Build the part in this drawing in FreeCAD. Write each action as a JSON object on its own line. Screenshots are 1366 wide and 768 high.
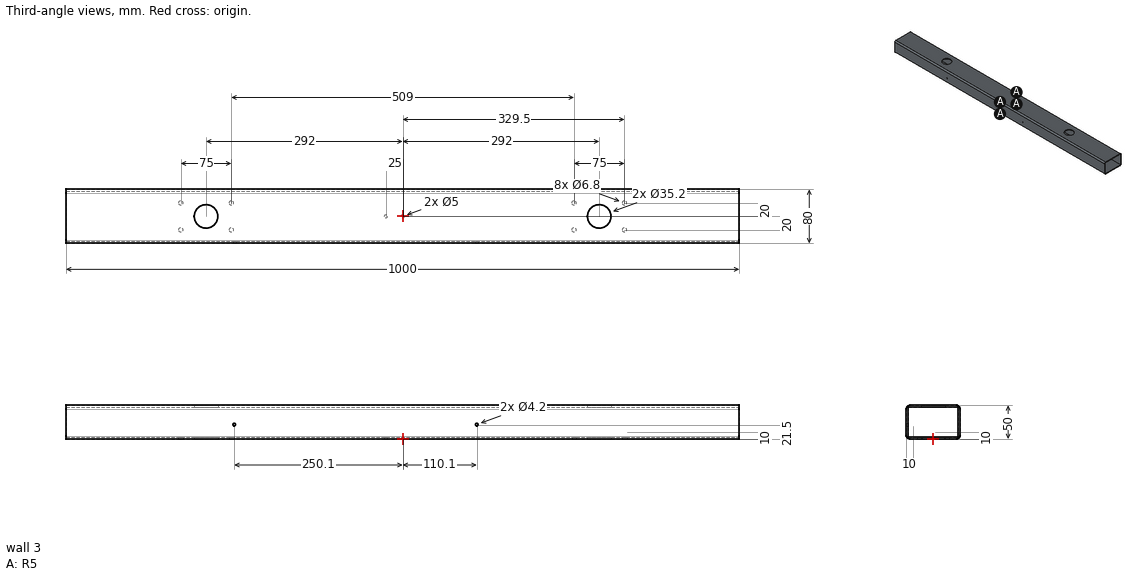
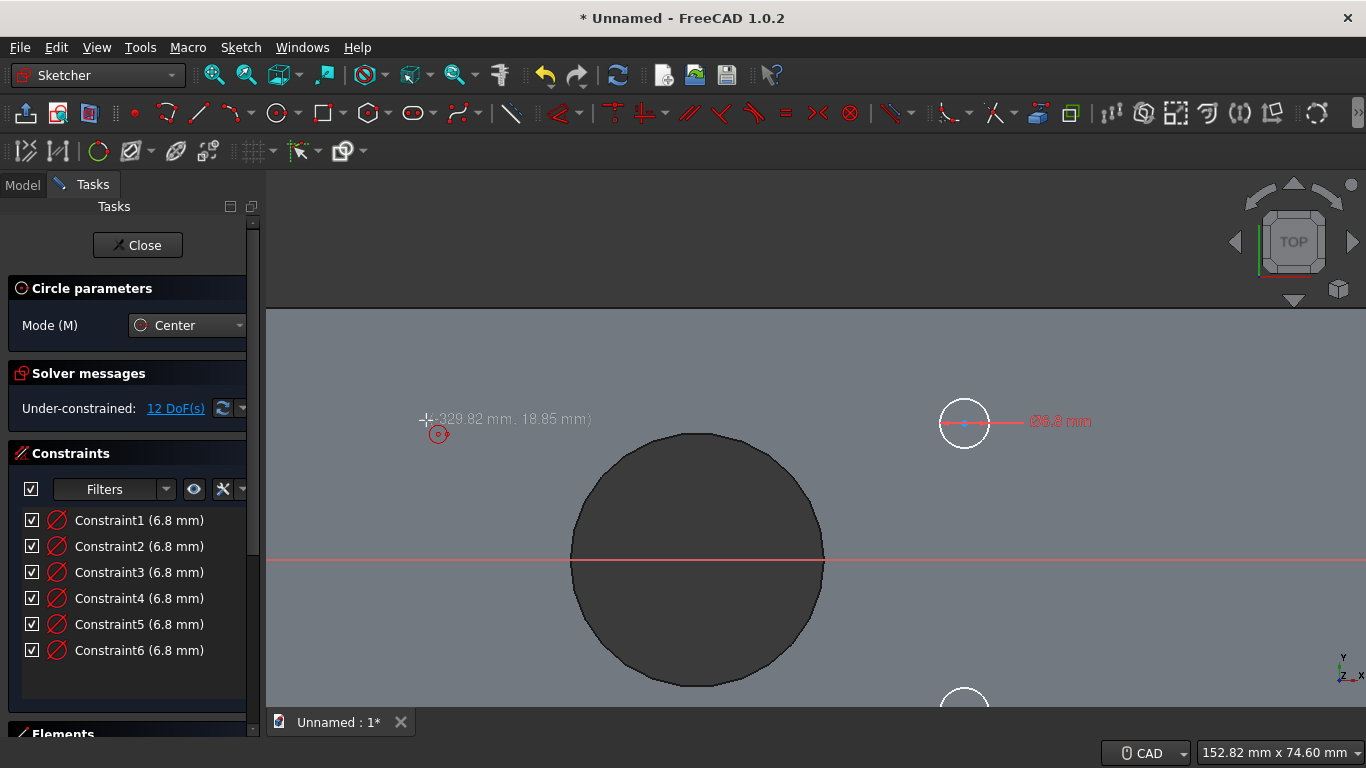
{"action": "scroll", "coordinate": [426, 419], "scroll_direction": "down", "scroll_amount": 10}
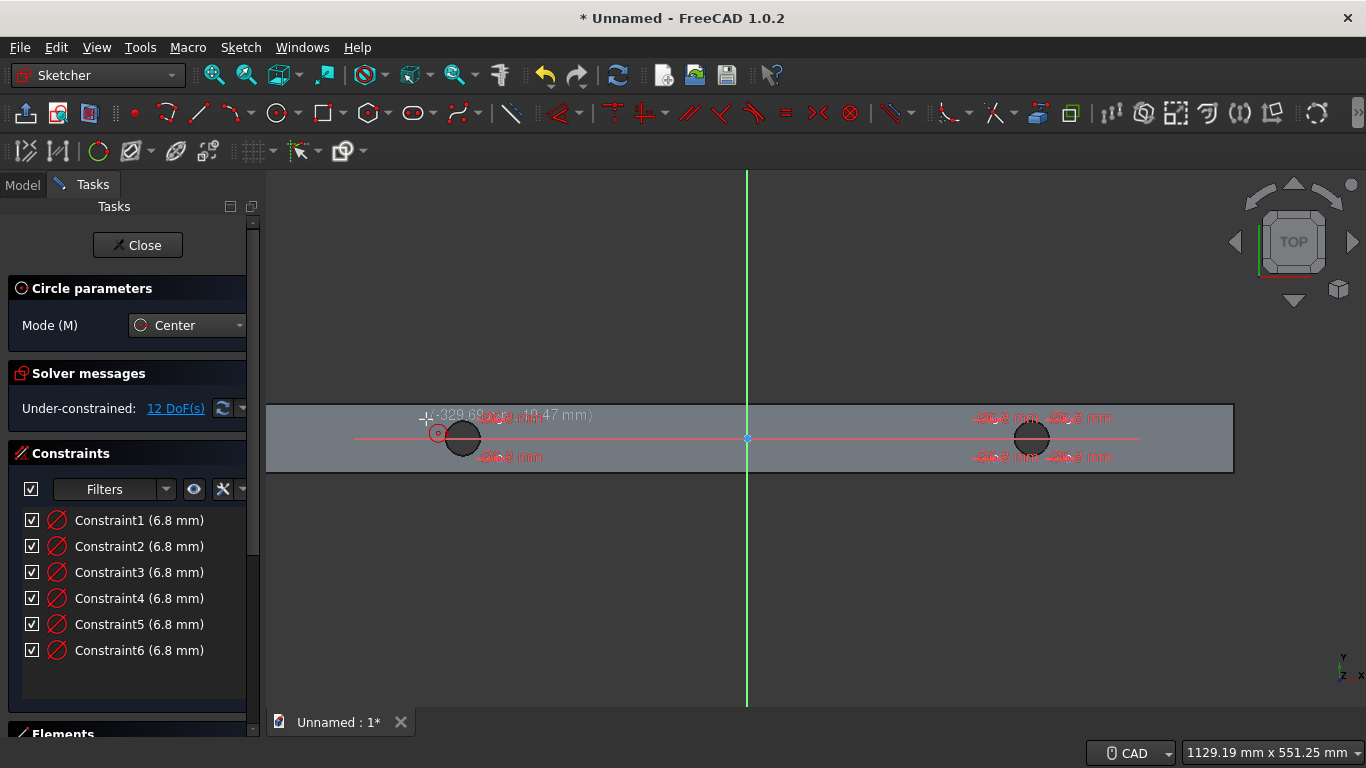
{"action": "left_click", "coordinate": [426, 419]}
{"action": "mouse_move", "coordinate": [429, 417]}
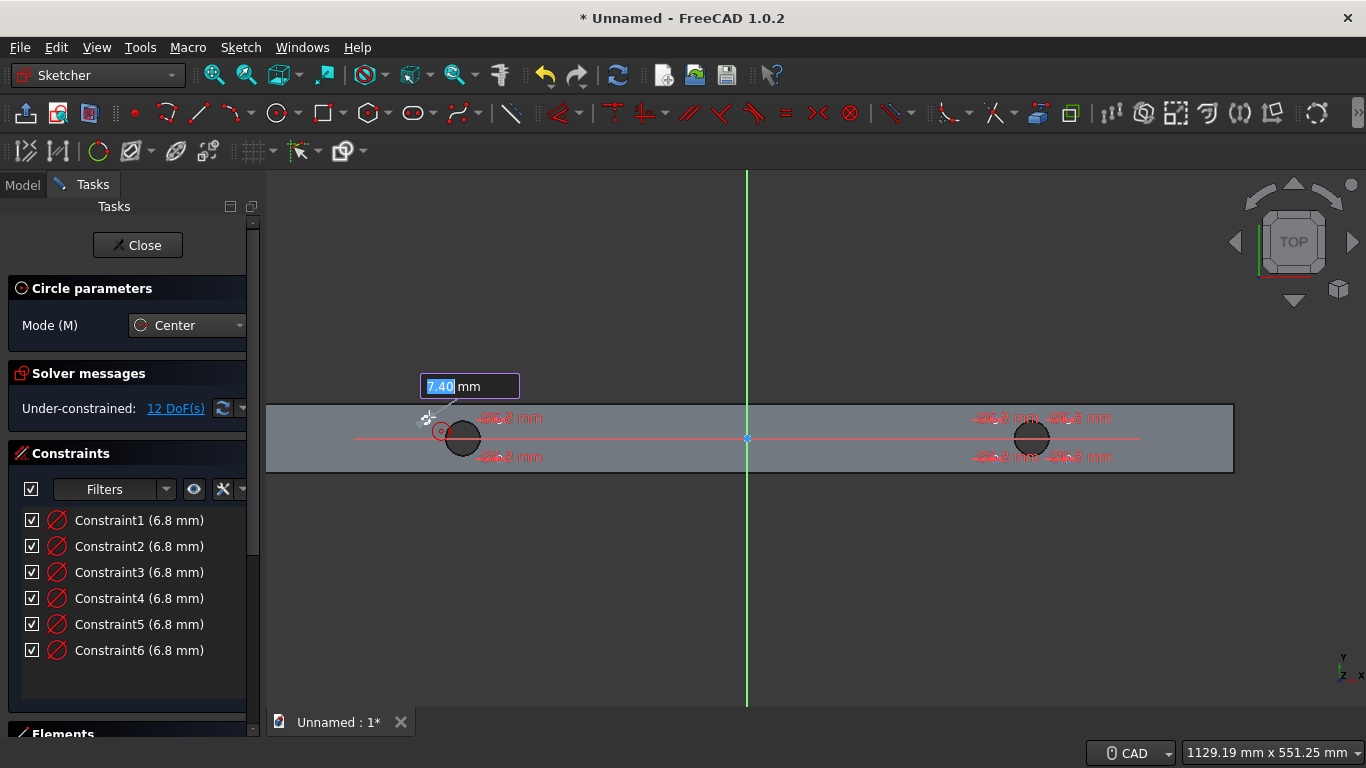
{"action": "type", "text": "6.8"}
{"action": "key", "text": "Return"}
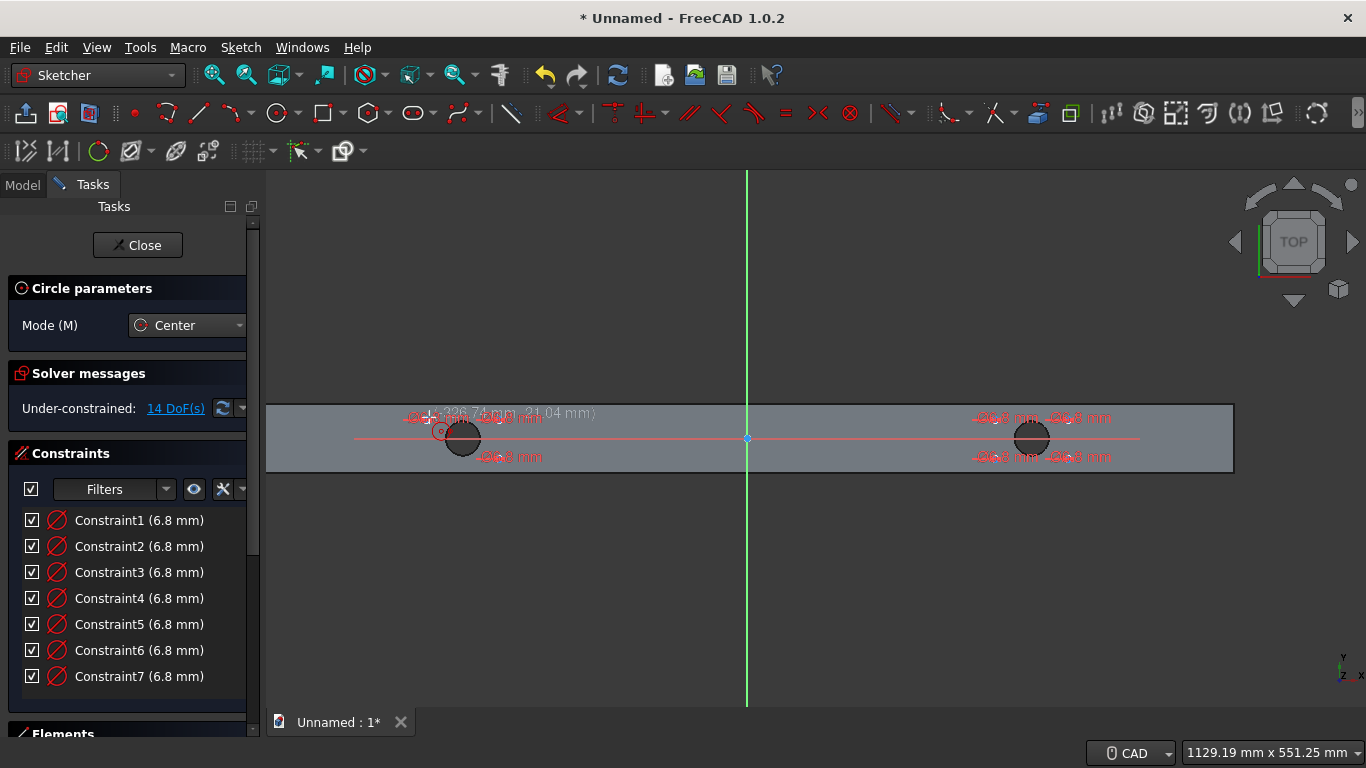
{"action": "scroll", "coordinate": [426, 458], "scroll_direction": "up", "scroll_amount": 10}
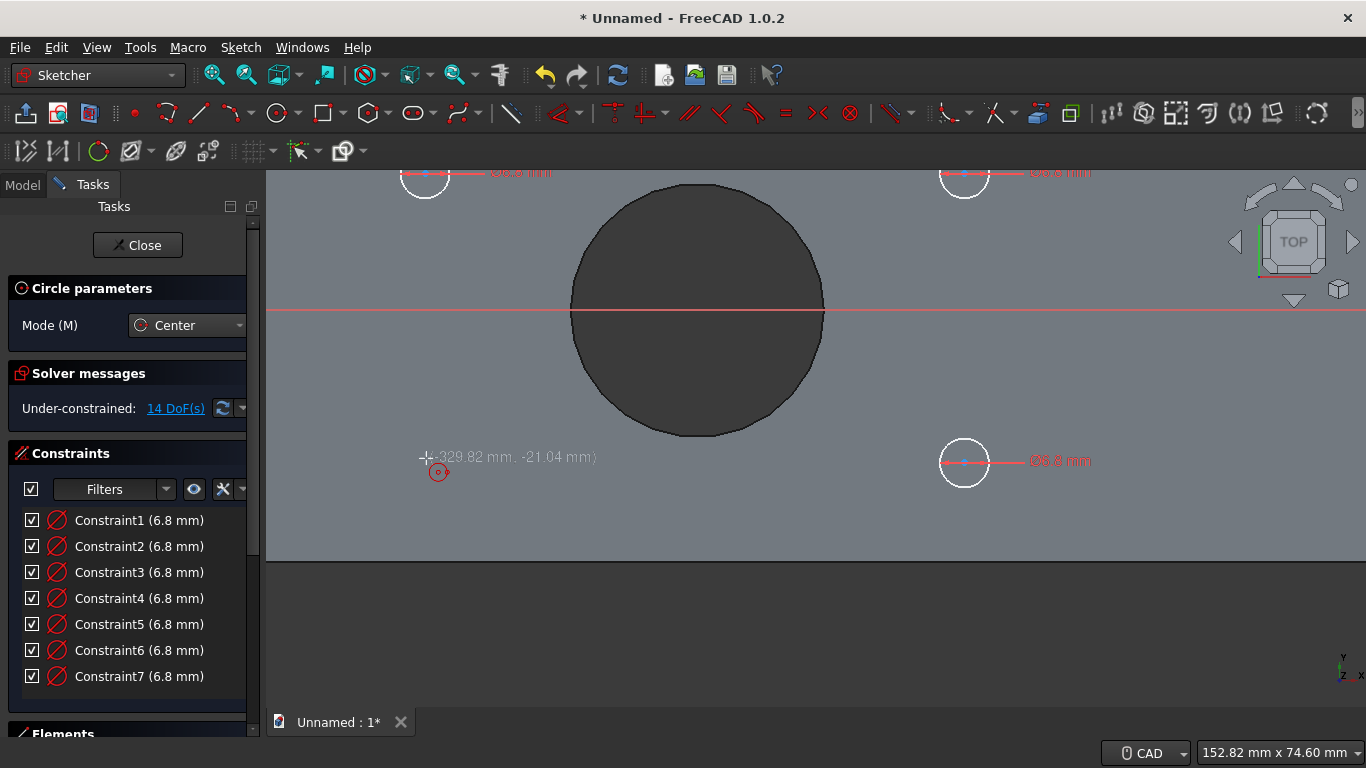
{"action": "scroll", "coordinate": [426, 459], "scroll_direction": "down", "scroll_amount": 10}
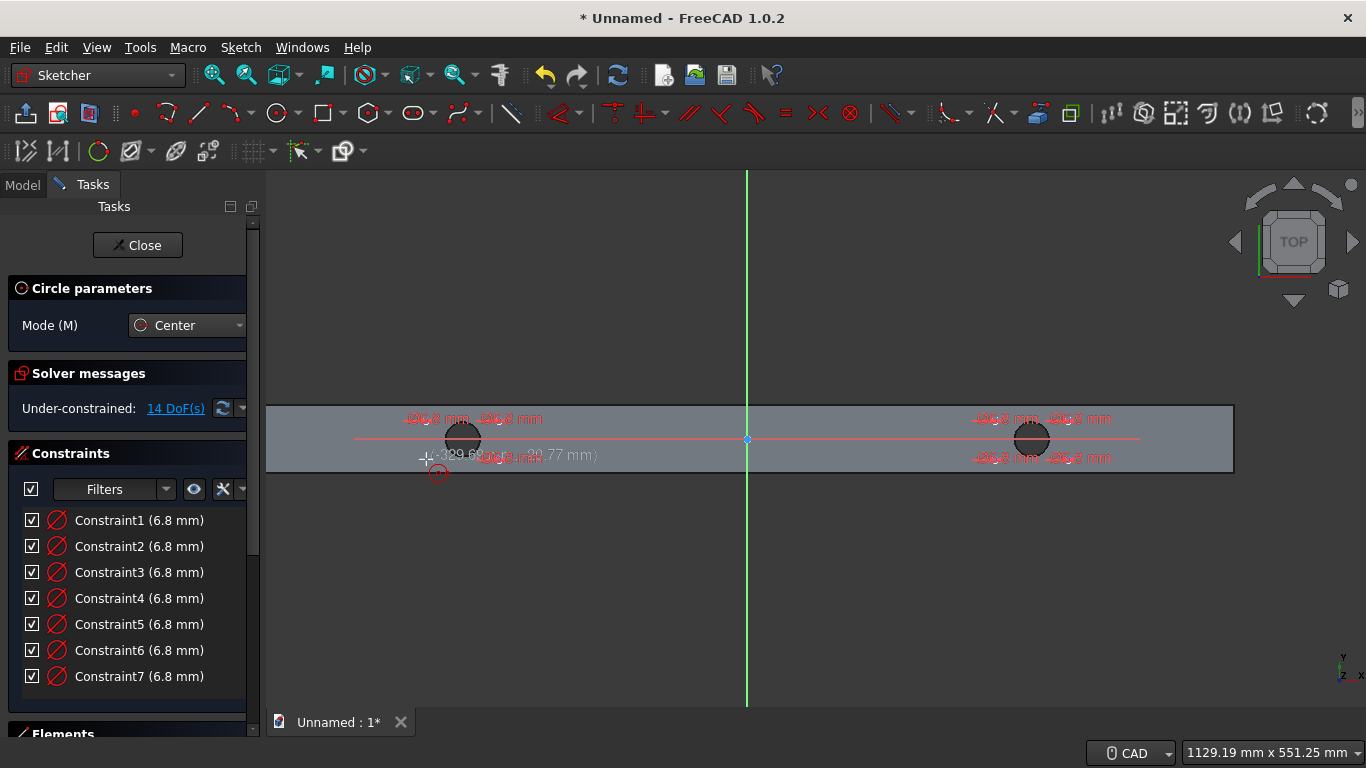
{"action": "left_click", "coordinate": [426, 459]}
{"action": "mouse_move", "coordinate": [429, 457]}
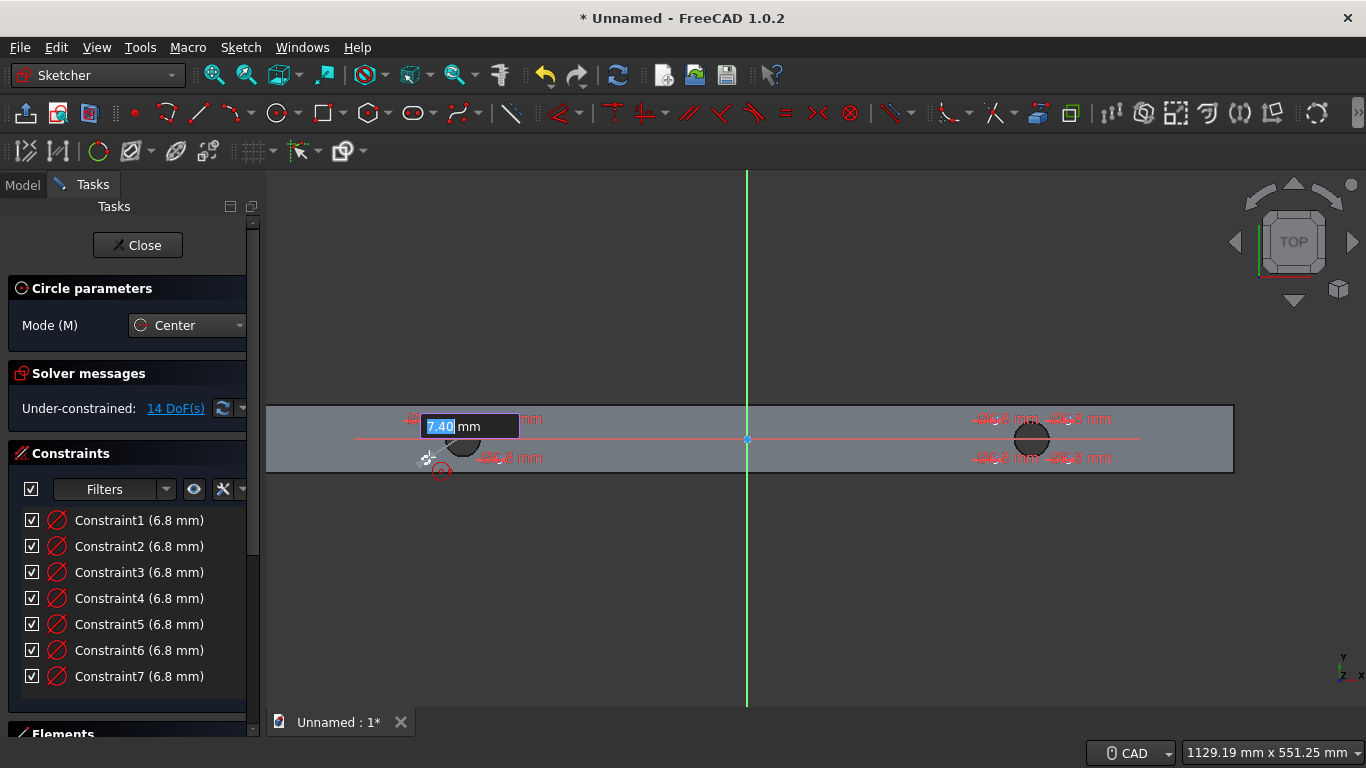
{"action": "type", "text": "6.8"}
{"action": "key", "text": "Return"}
{"action": "key", "text": "Escape"}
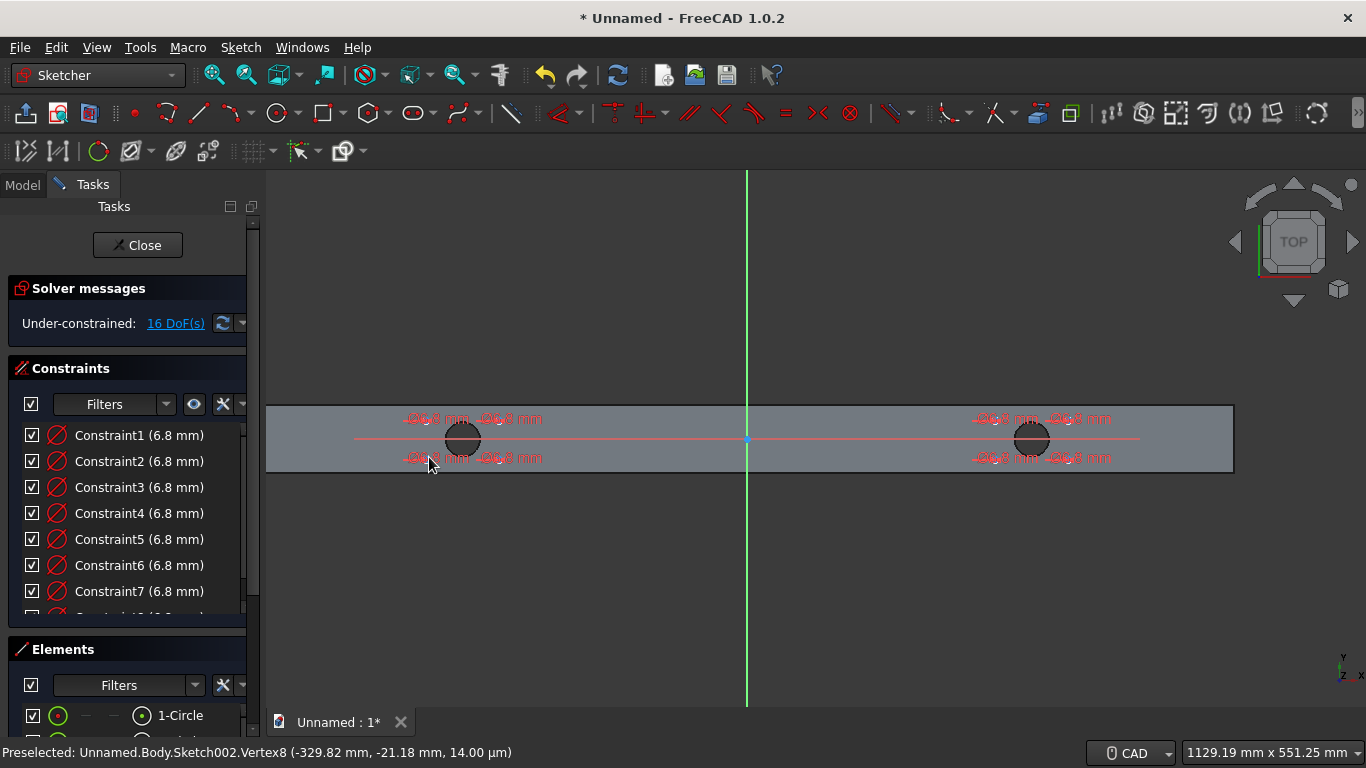
{"action": "left_click", "coordinate": [1068, 421]}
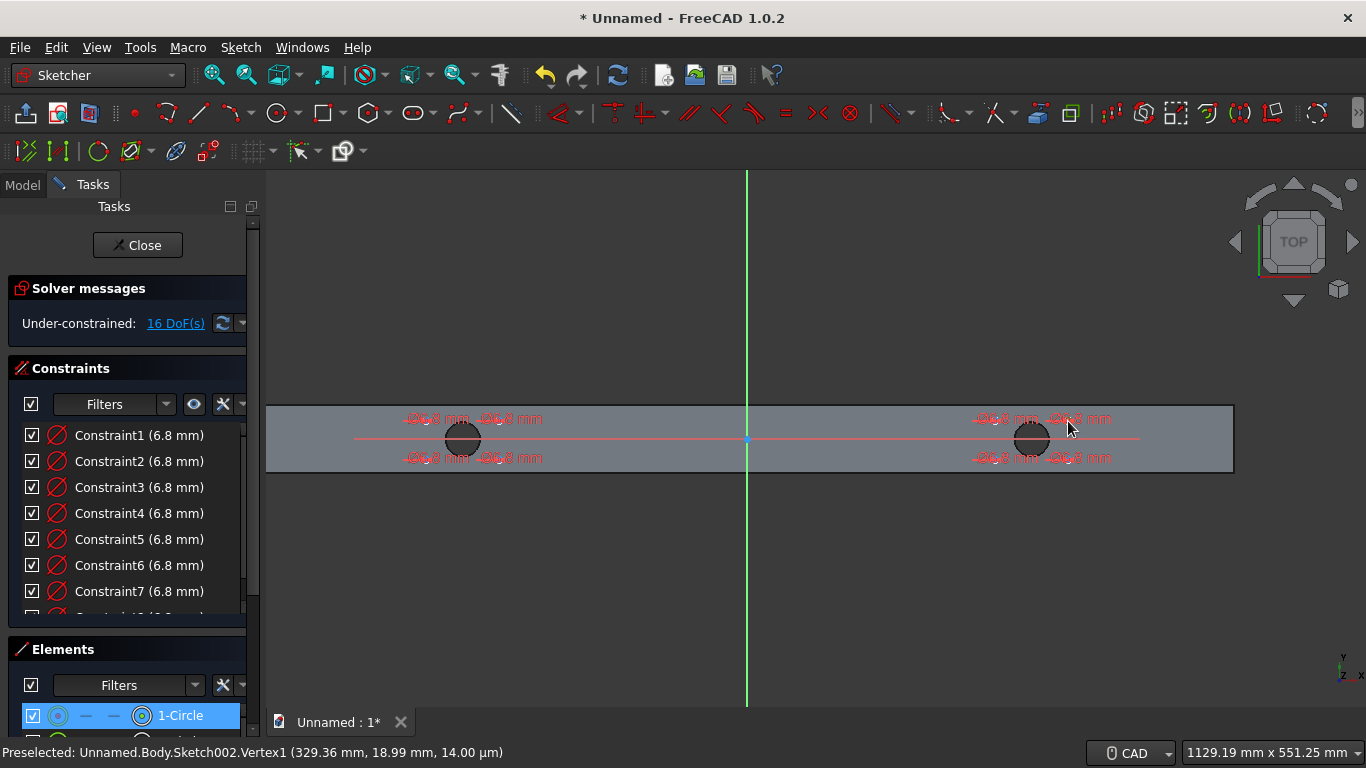
{"action": "left_click", "coordinate": [1068, 460]}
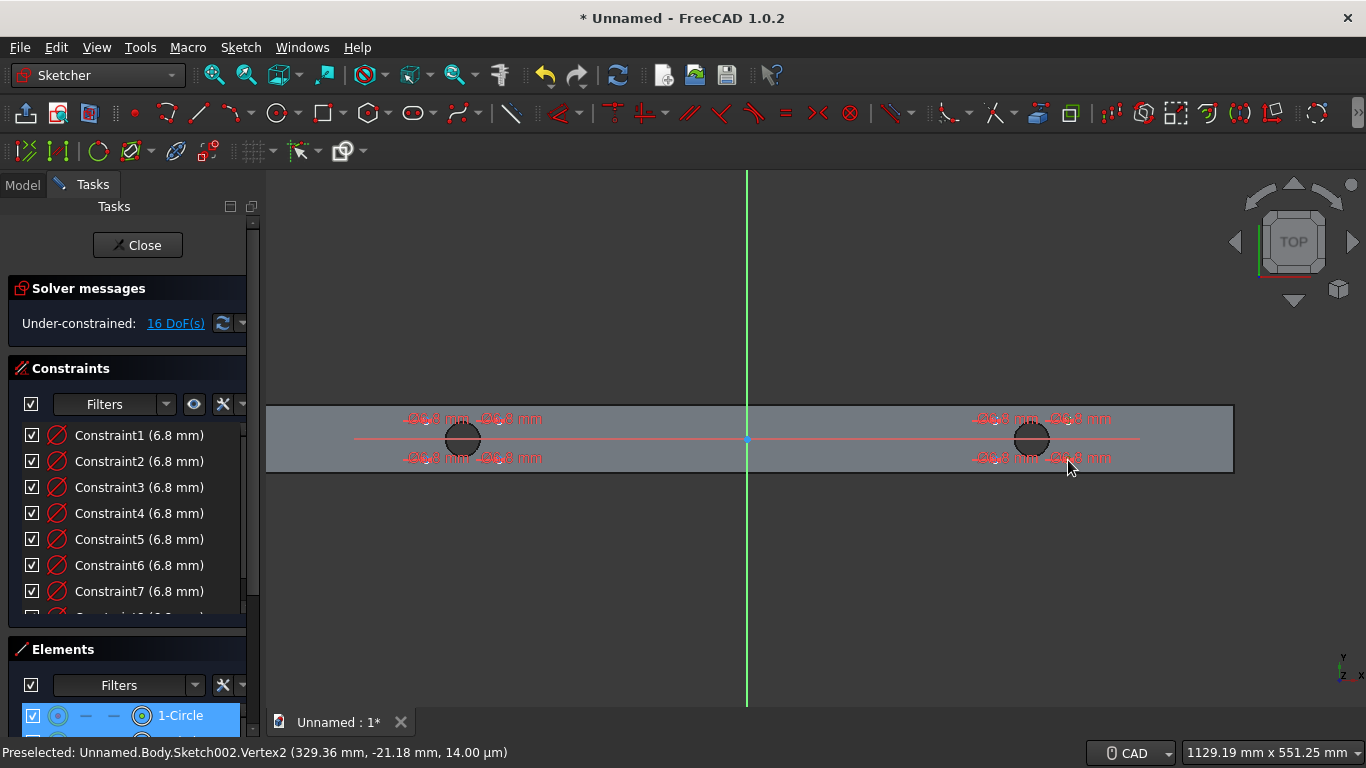
{"action": "left_click", "coordinate": [668, 114]}